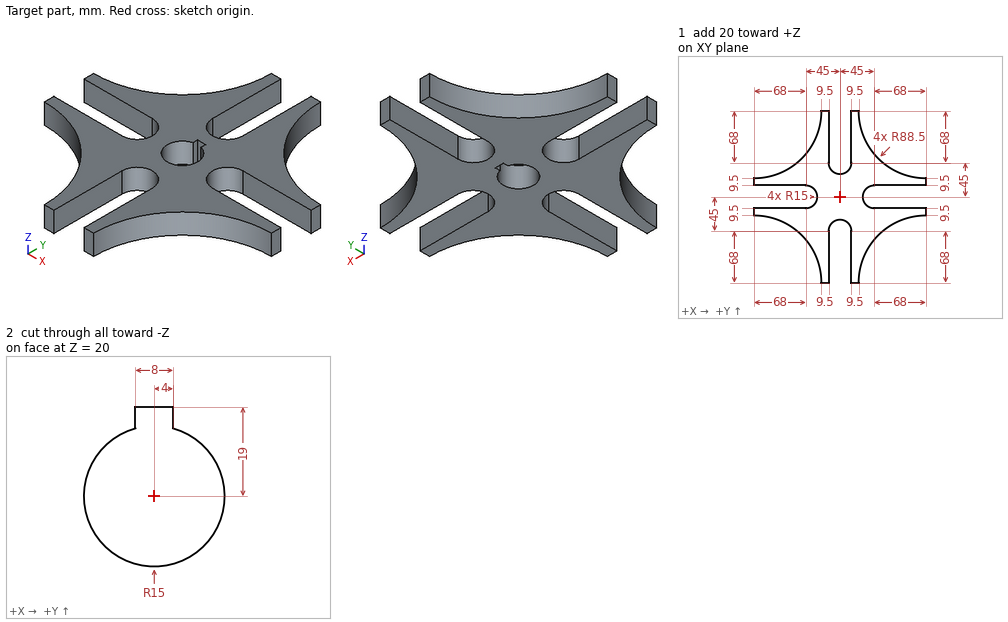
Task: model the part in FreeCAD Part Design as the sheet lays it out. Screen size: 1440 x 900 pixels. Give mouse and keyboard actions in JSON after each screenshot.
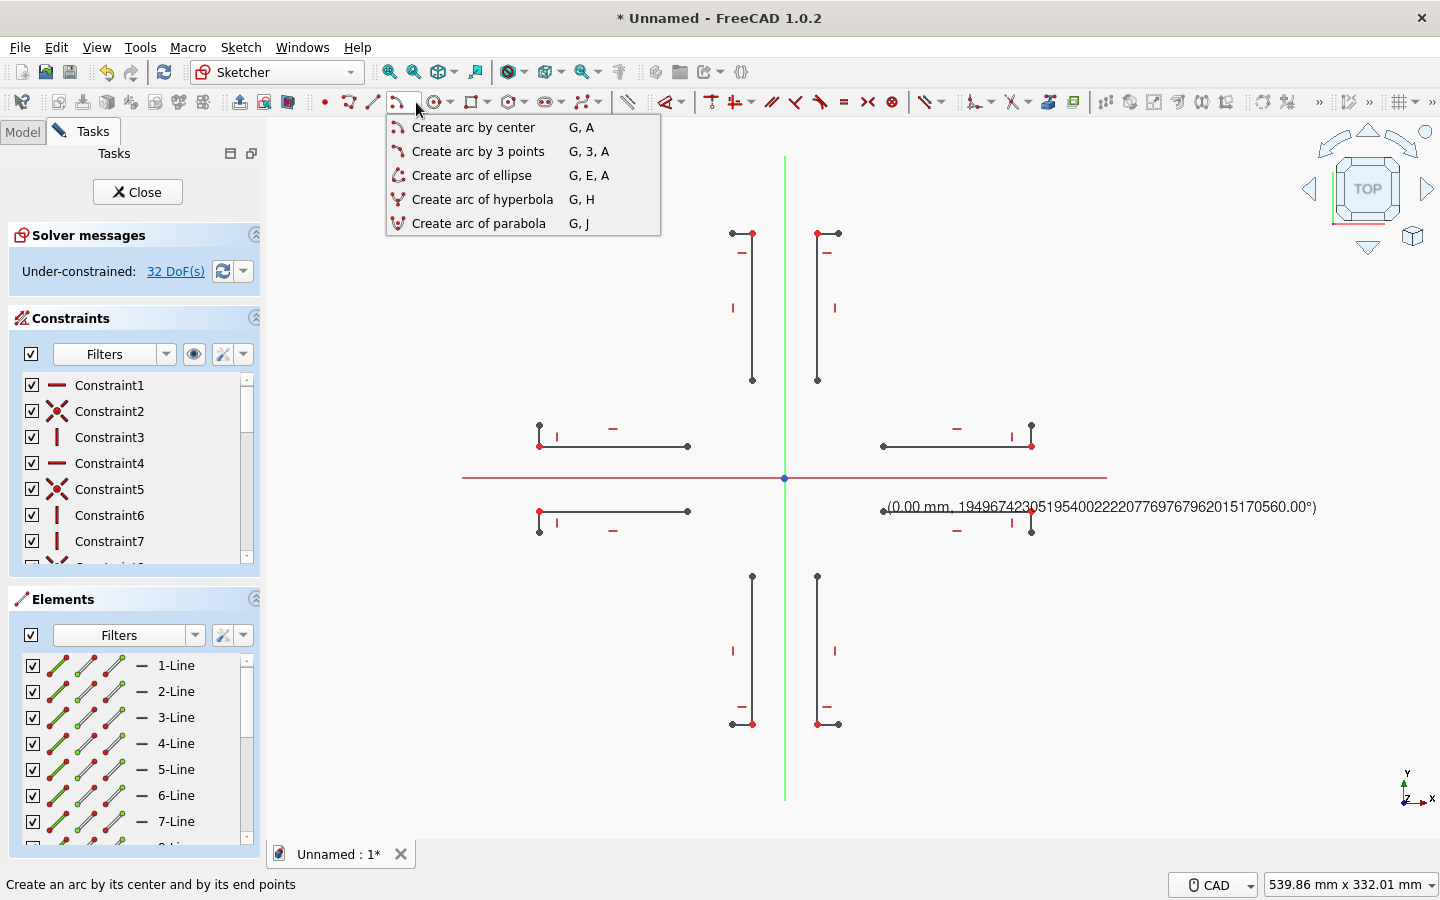
{"action": "left_click", "coordinate": [524, 151]}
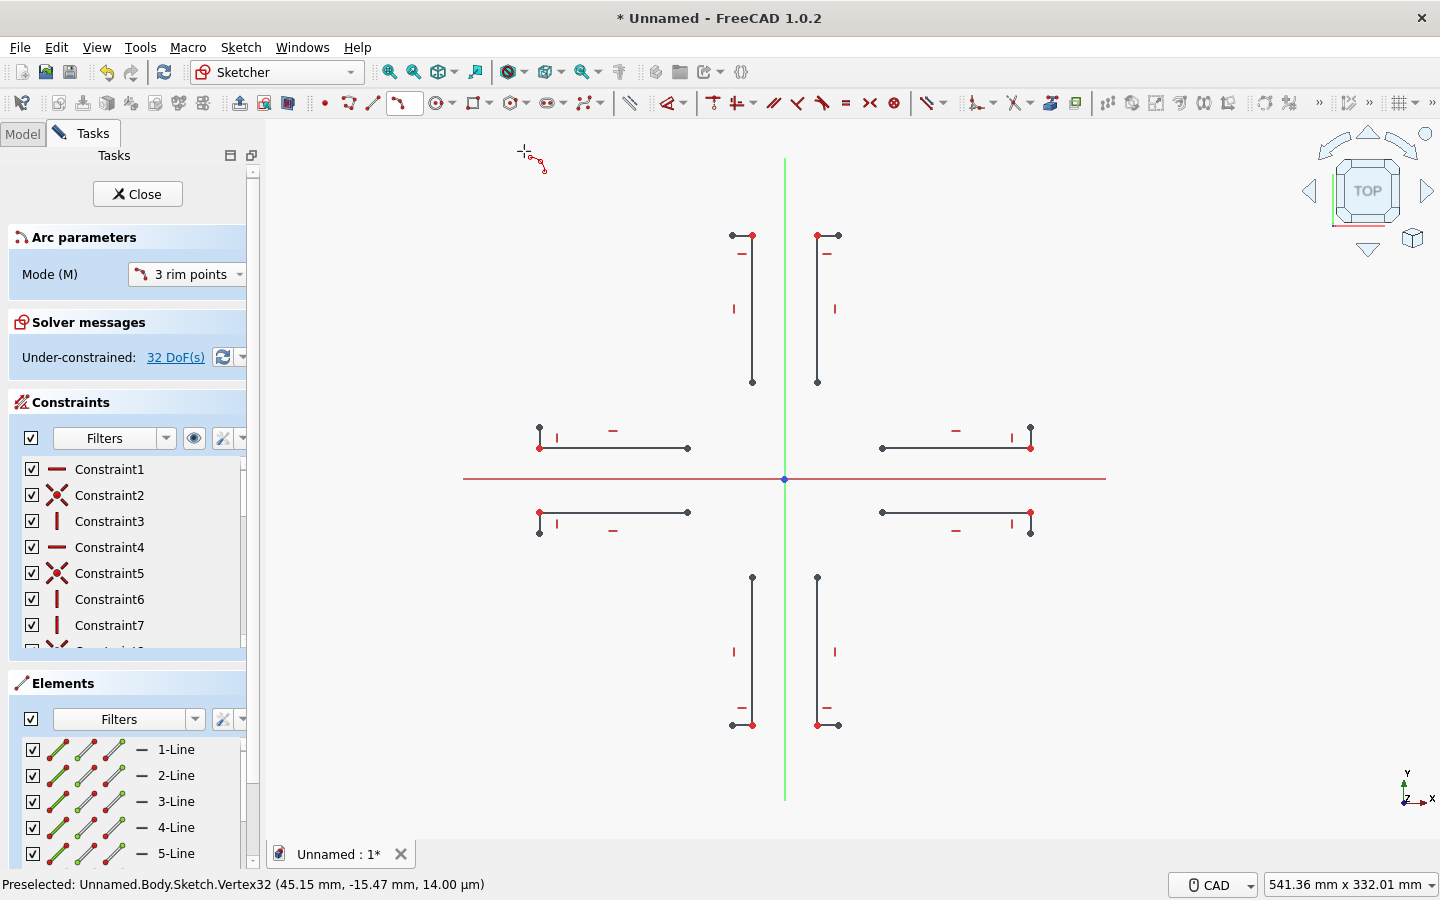
{"action": "scroll", "coordinate": [1030, 426], "scroll_direction": "up", "scroll_amount": 3}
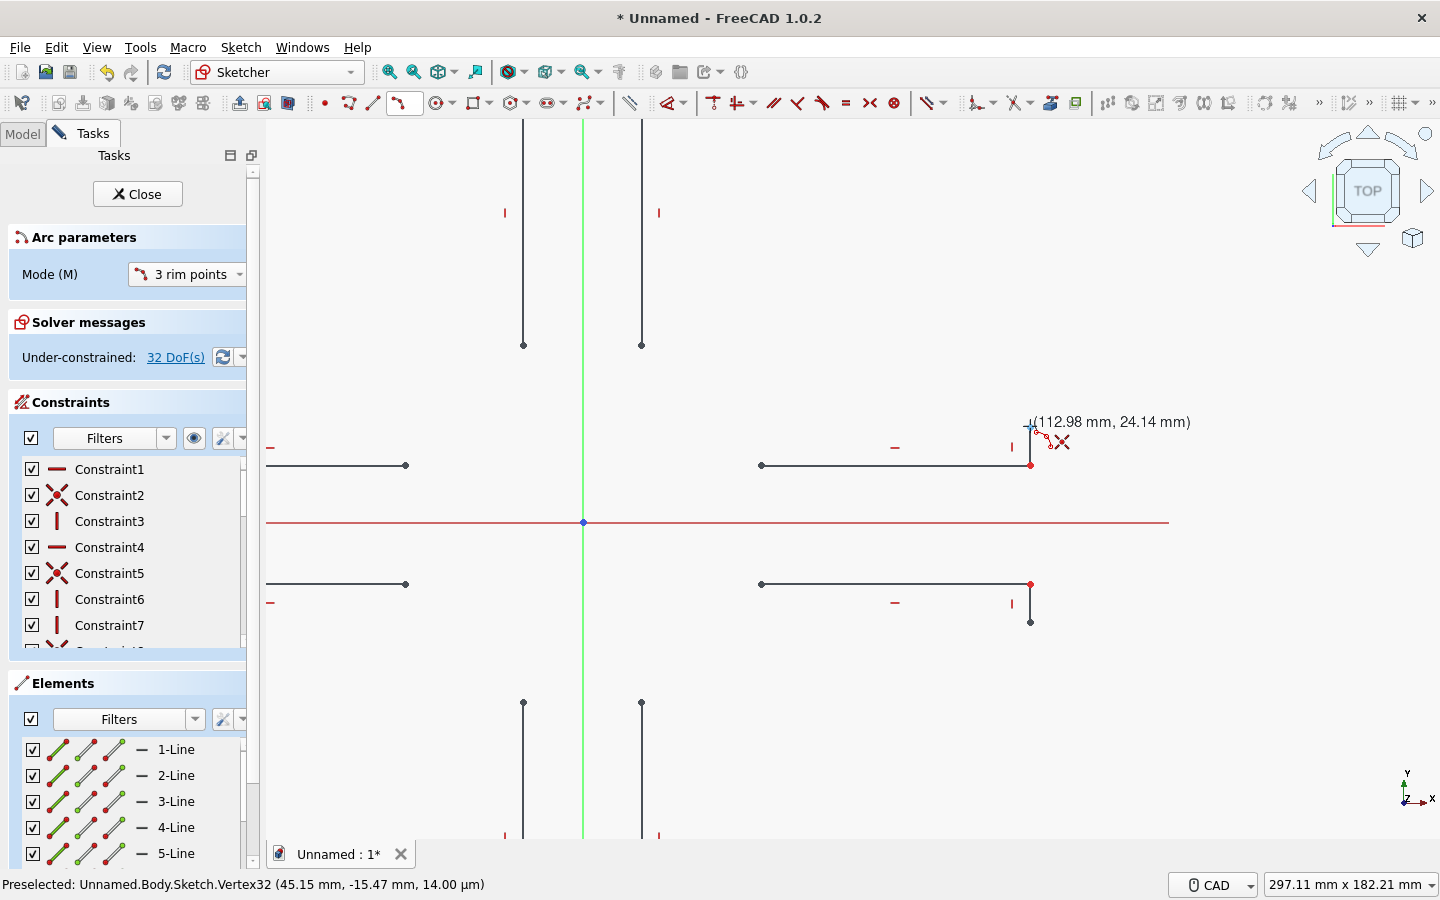
{"action": "left_click", "coordinate": [1030, 428]}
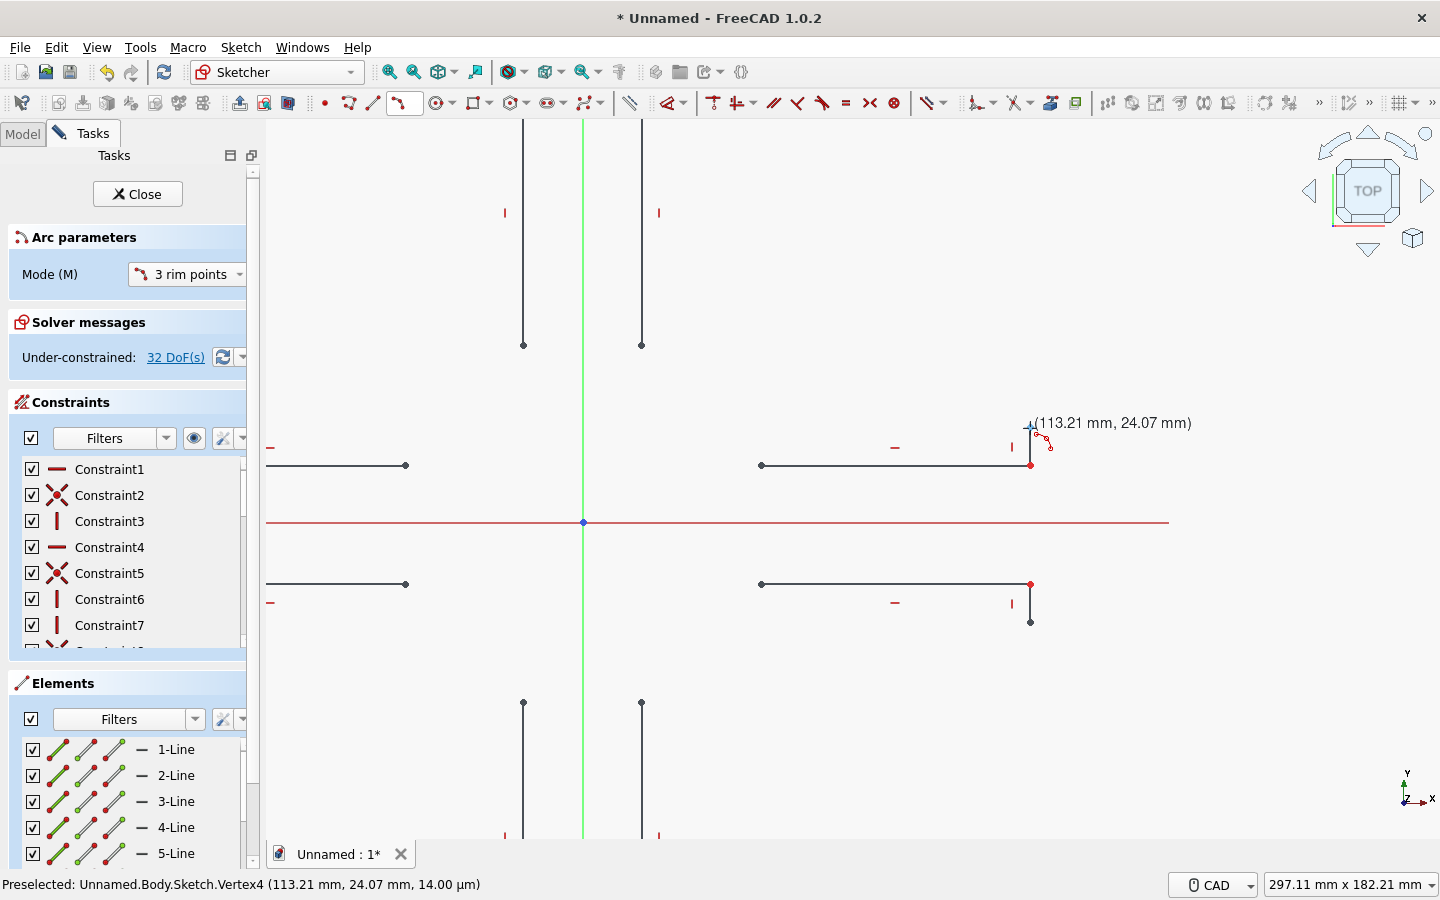
{"action": "scroll", "coordinate": [1030, 426], "scroll_direction": "down", "scroll_amount": 3}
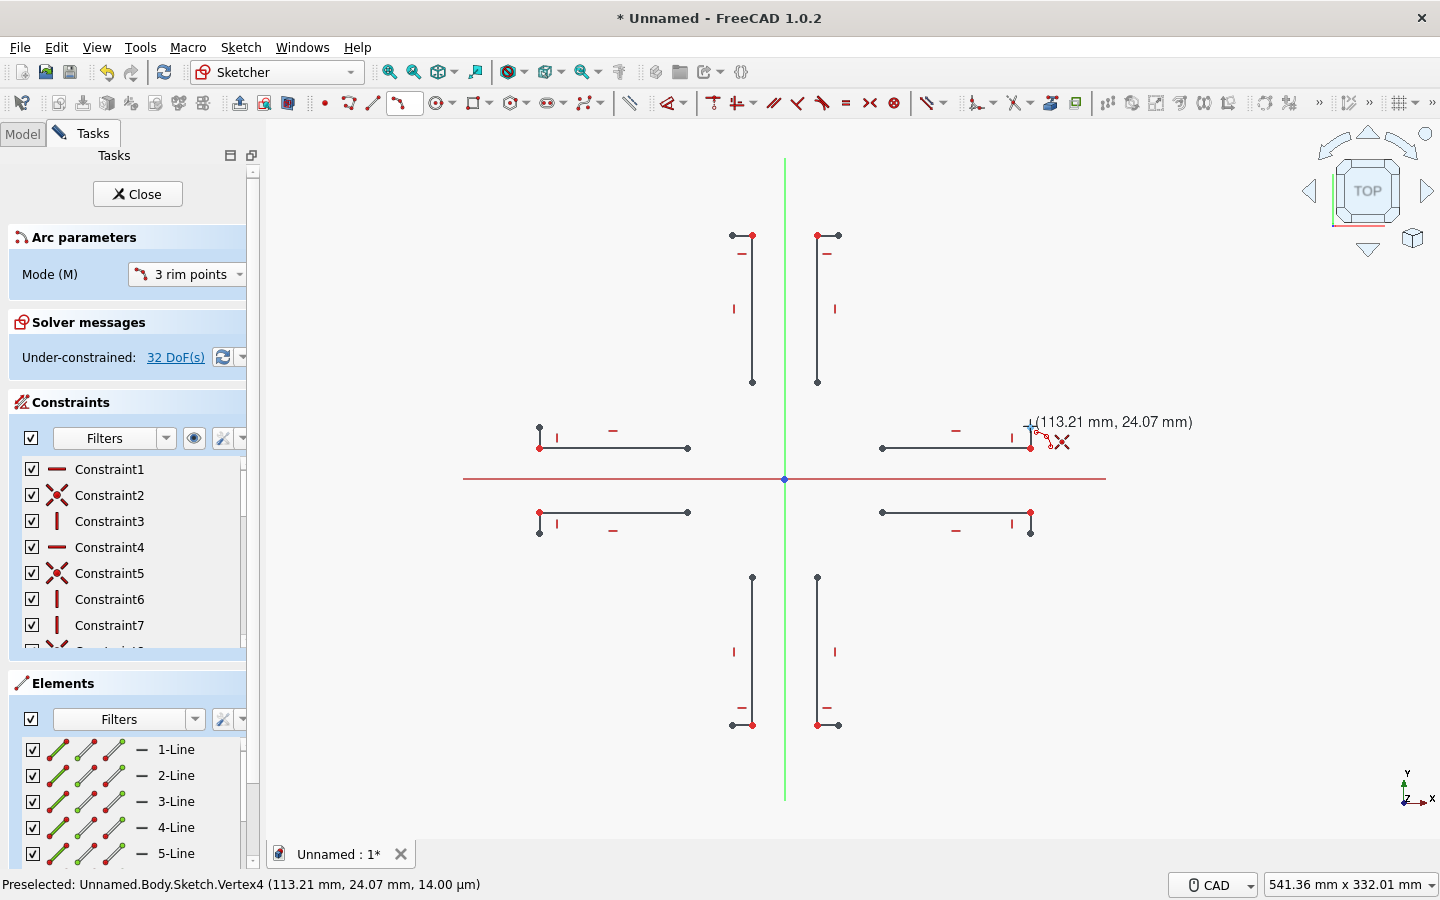
{"action": "scroll", "coordinate": [838, 234], "scroll_direction": "up", "scroll_amount": 3}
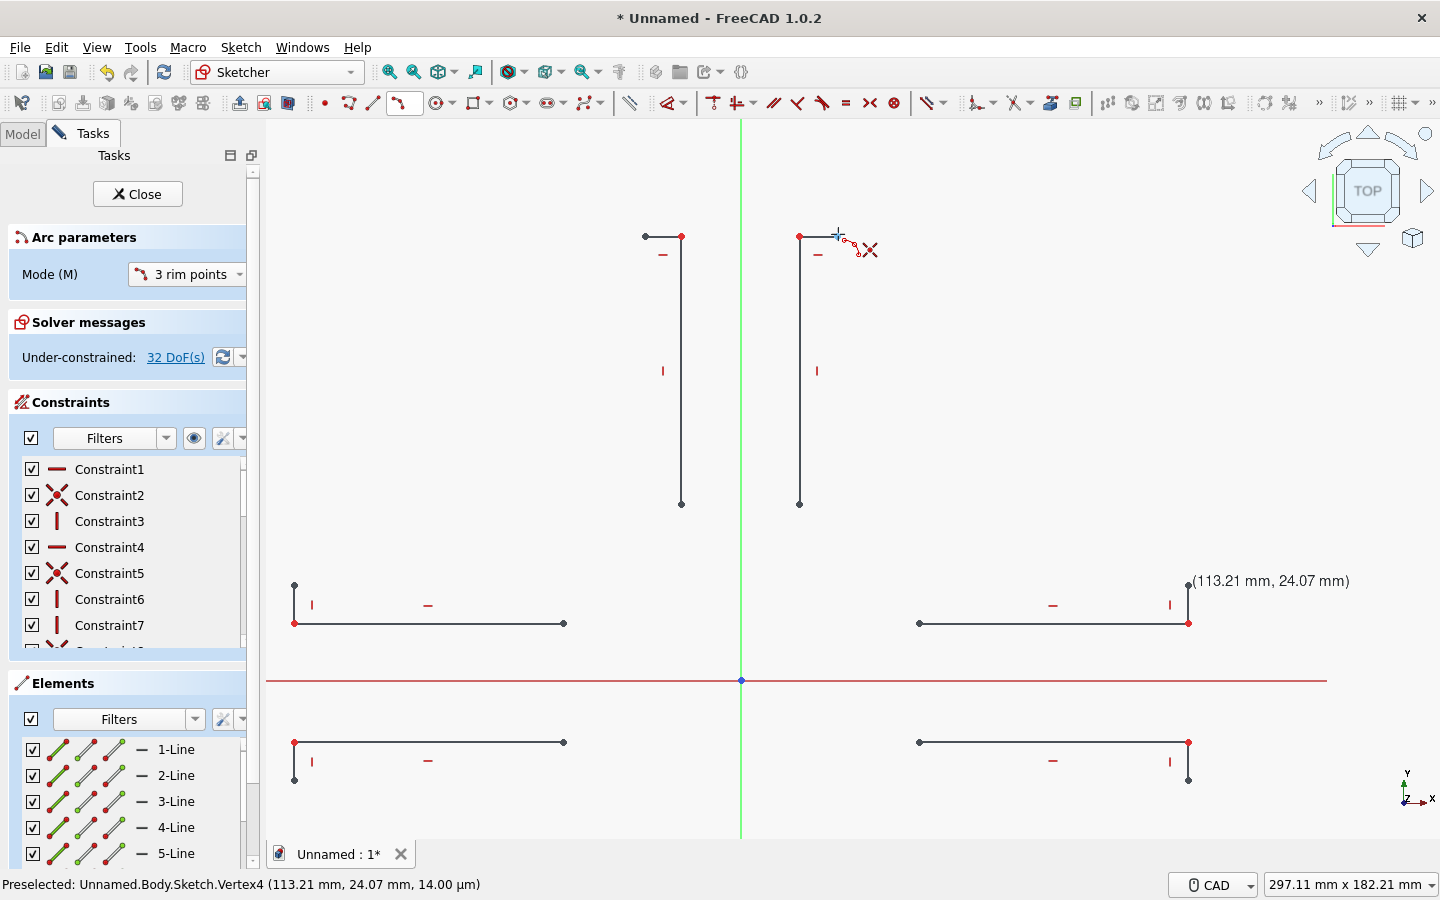
{"action": "left_click", "coordinate": [838, 237]}
{"action": "left_click", "coordinate": [940, 482]}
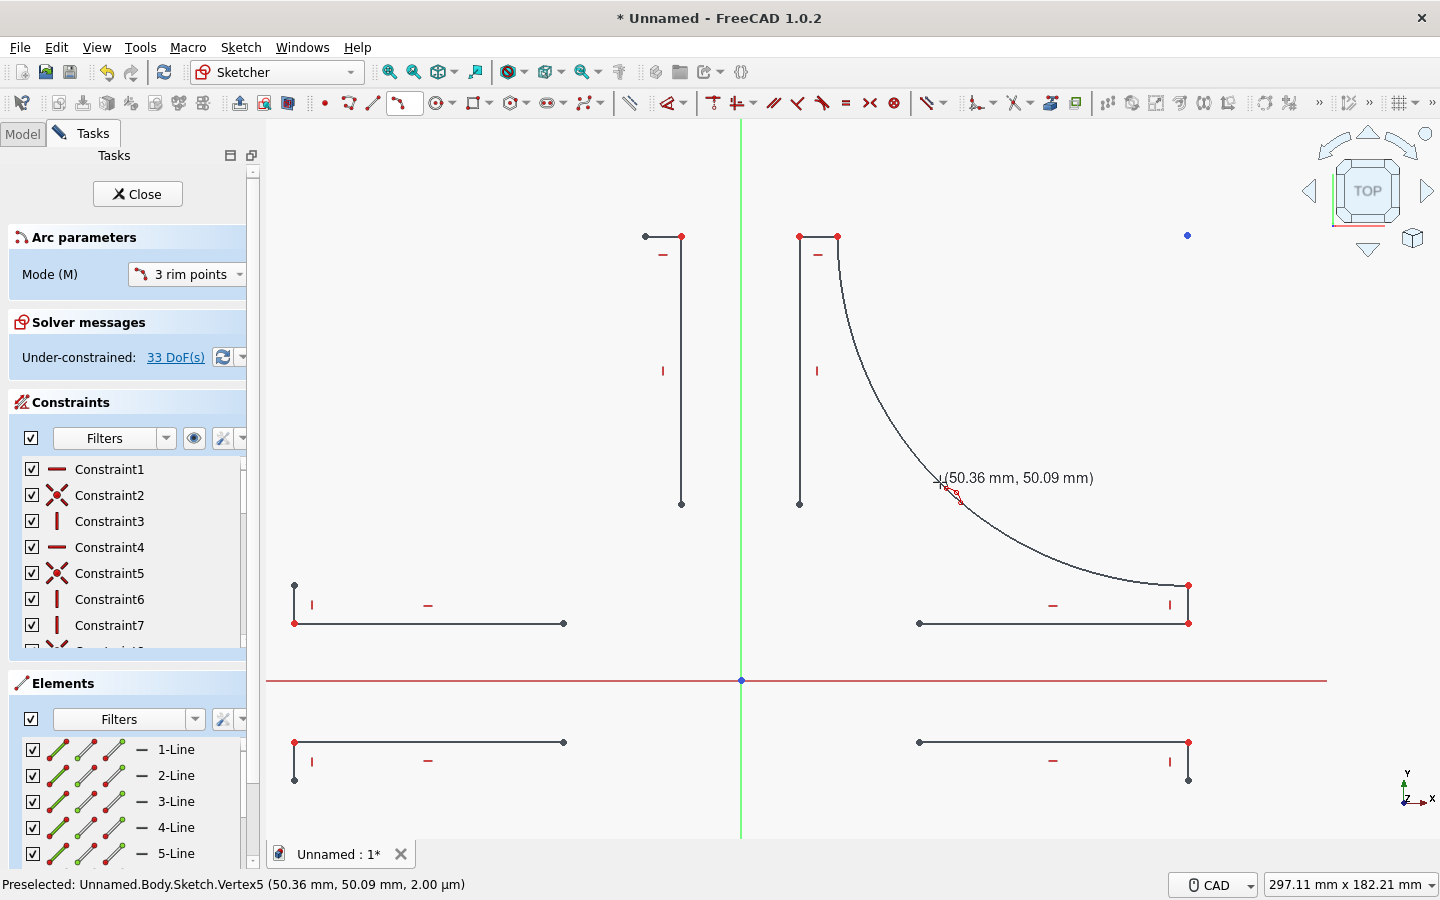
{"action": "left_click", "coordinate": [800, 504]}
{"action": "left_click", "coordinate": [681, 504]}
{"action": "left_click", "coordinate": [706, 551]}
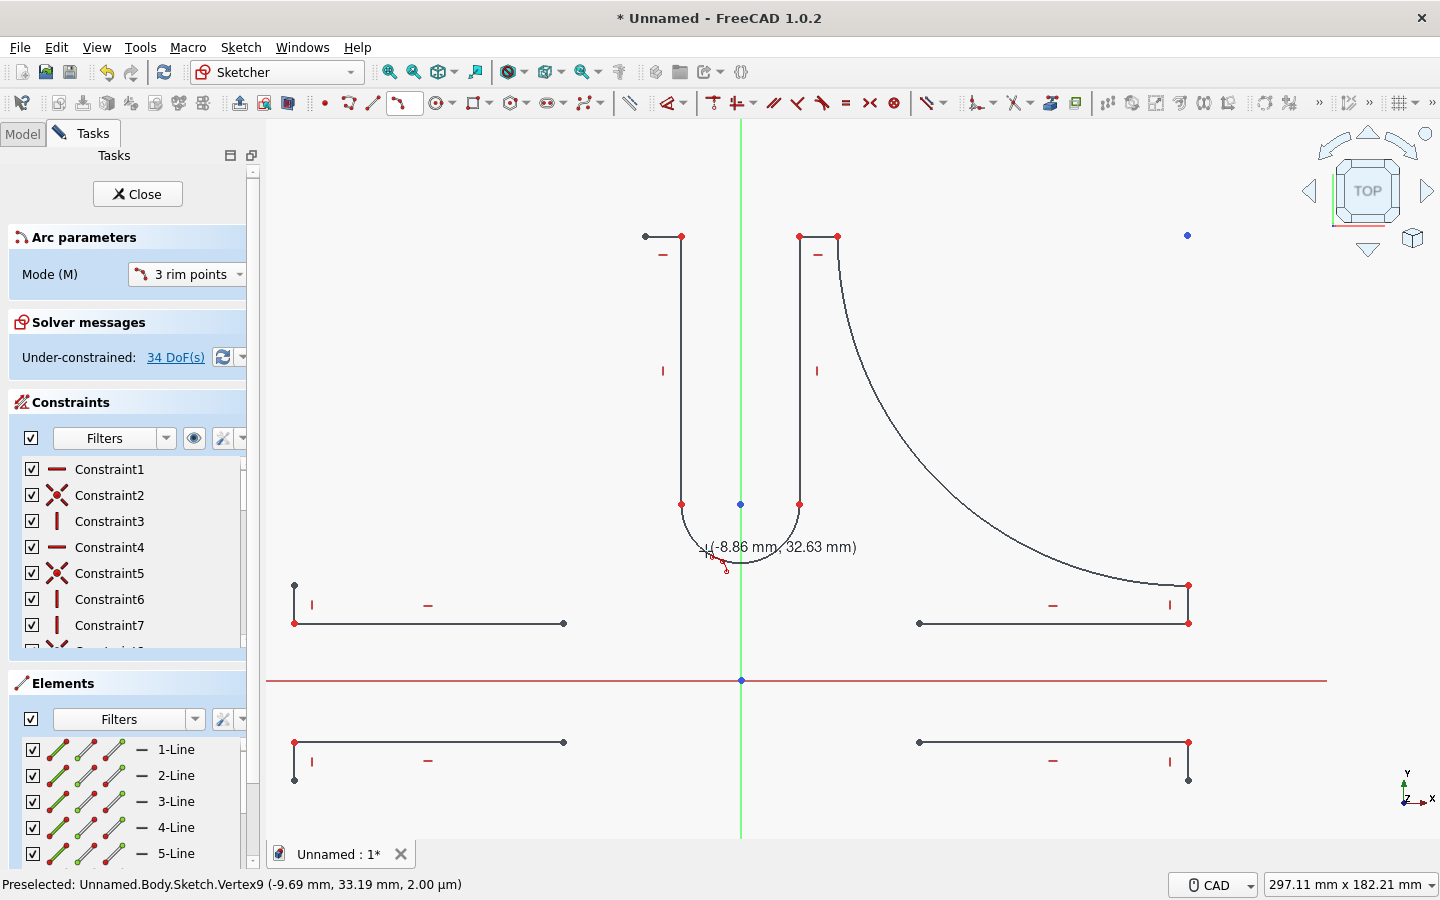
{"action": "left_click", "coordinate": [645, 237]}
{"action": "left_click", "coordinate": [294, 586]}
{"action": "left_click", "coordinate": [542, 482]}